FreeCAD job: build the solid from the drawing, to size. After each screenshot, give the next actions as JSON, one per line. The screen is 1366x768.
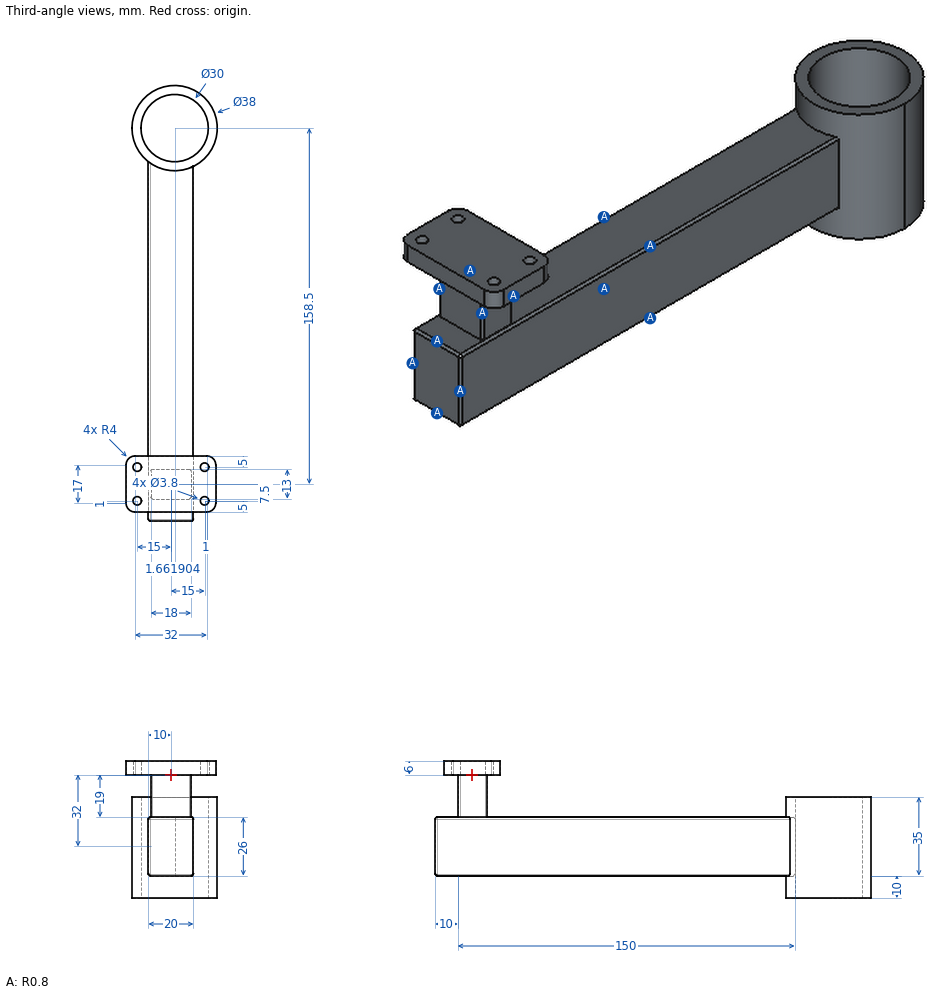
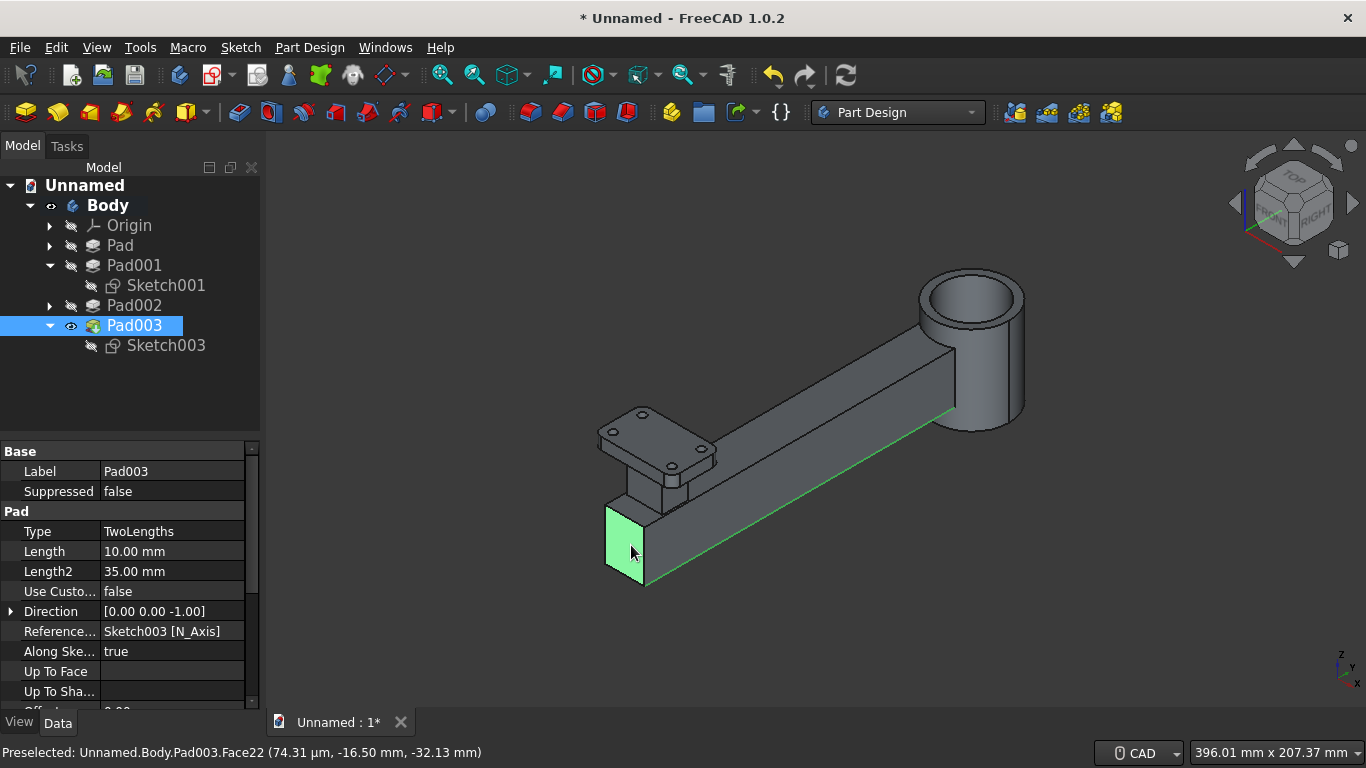
{"action": "left_click", "coordinate": [662, 492], "text": "ctrl"}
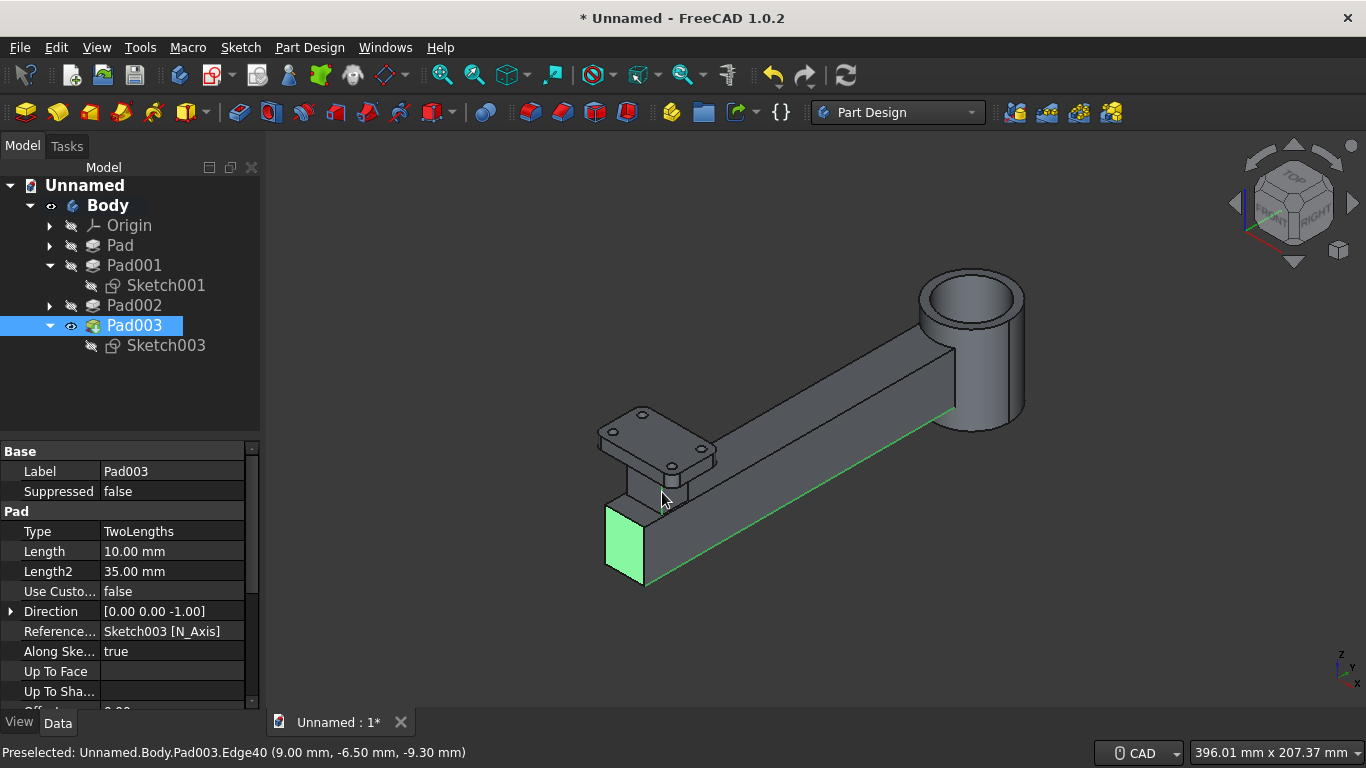
{"action": "left_click", "coordinate": [800, 437], "text": "ctrl"}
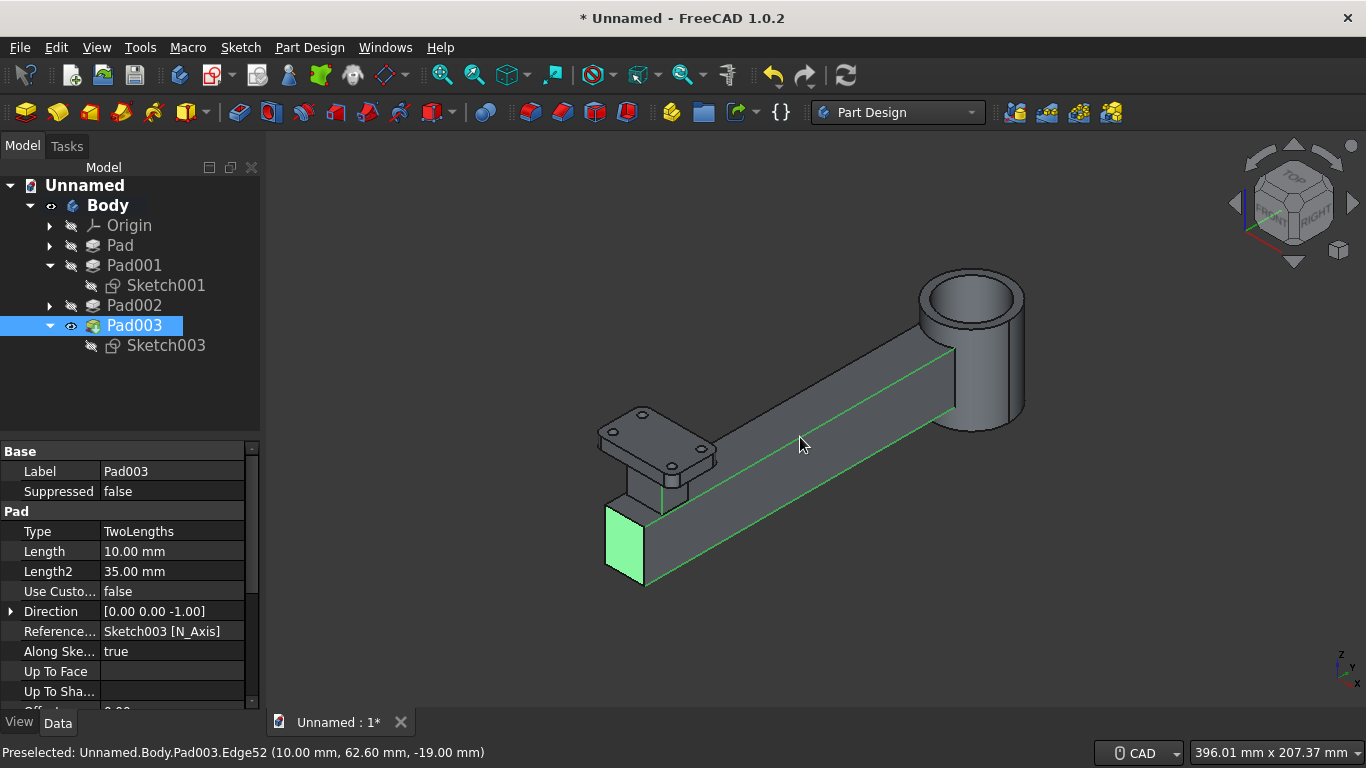
{"action": "key", "text": "2"}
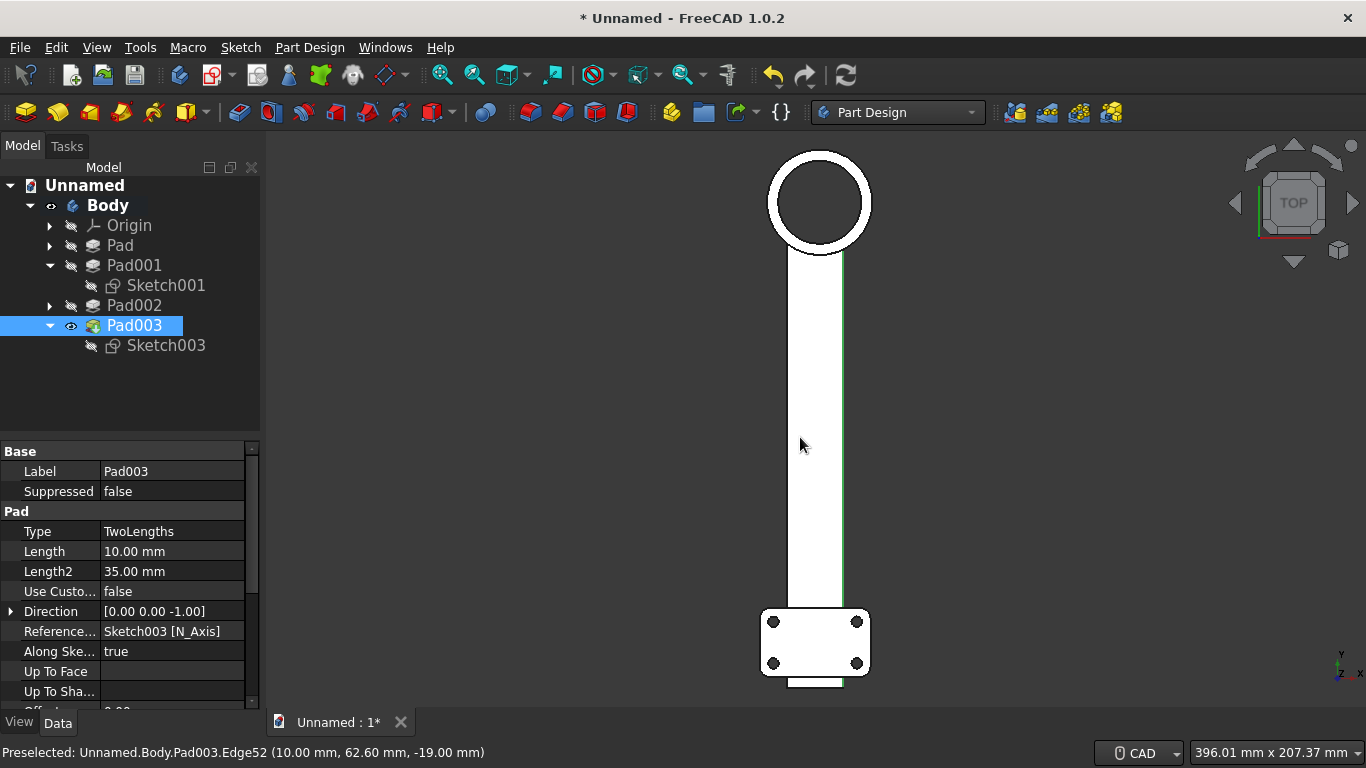
{"action": "left_click", "coordinate": [787, 465], "text": "ctrl"}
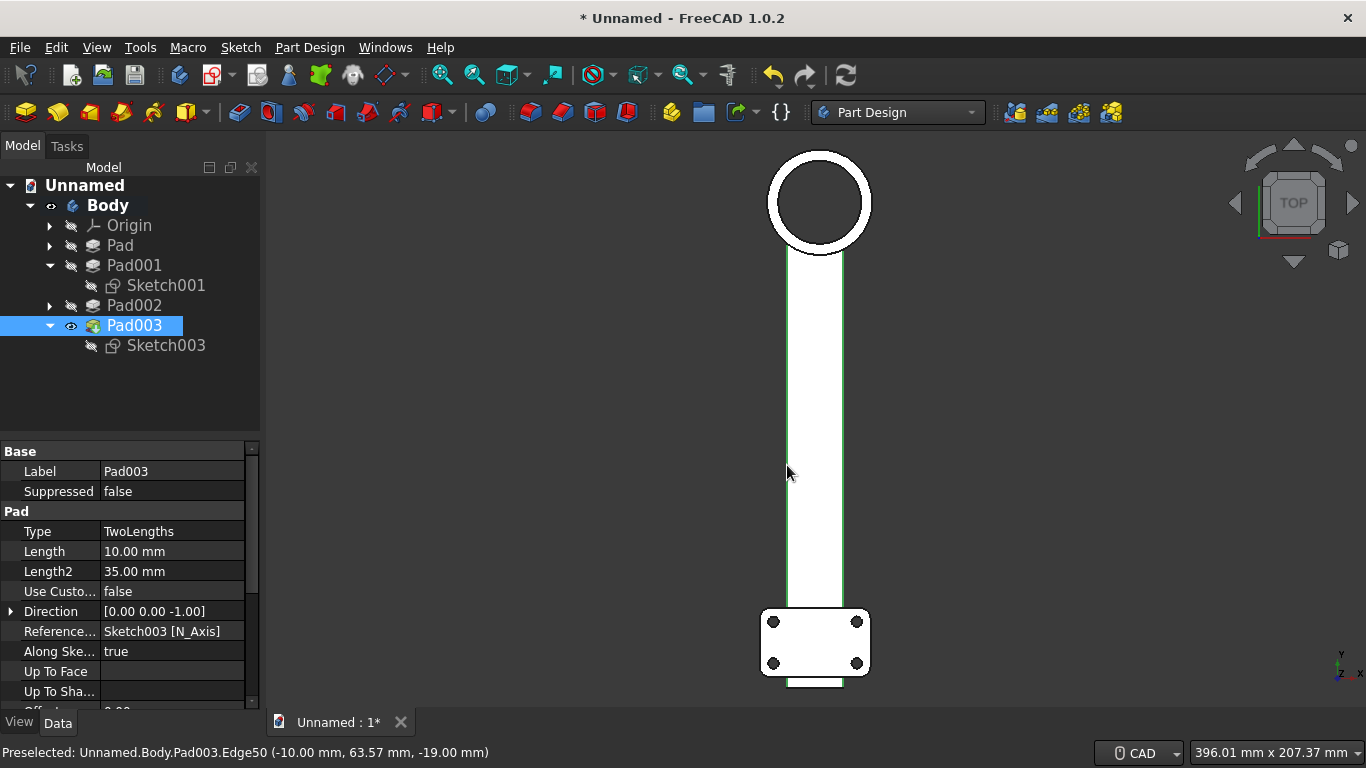
{"action": "key", "text": "1"}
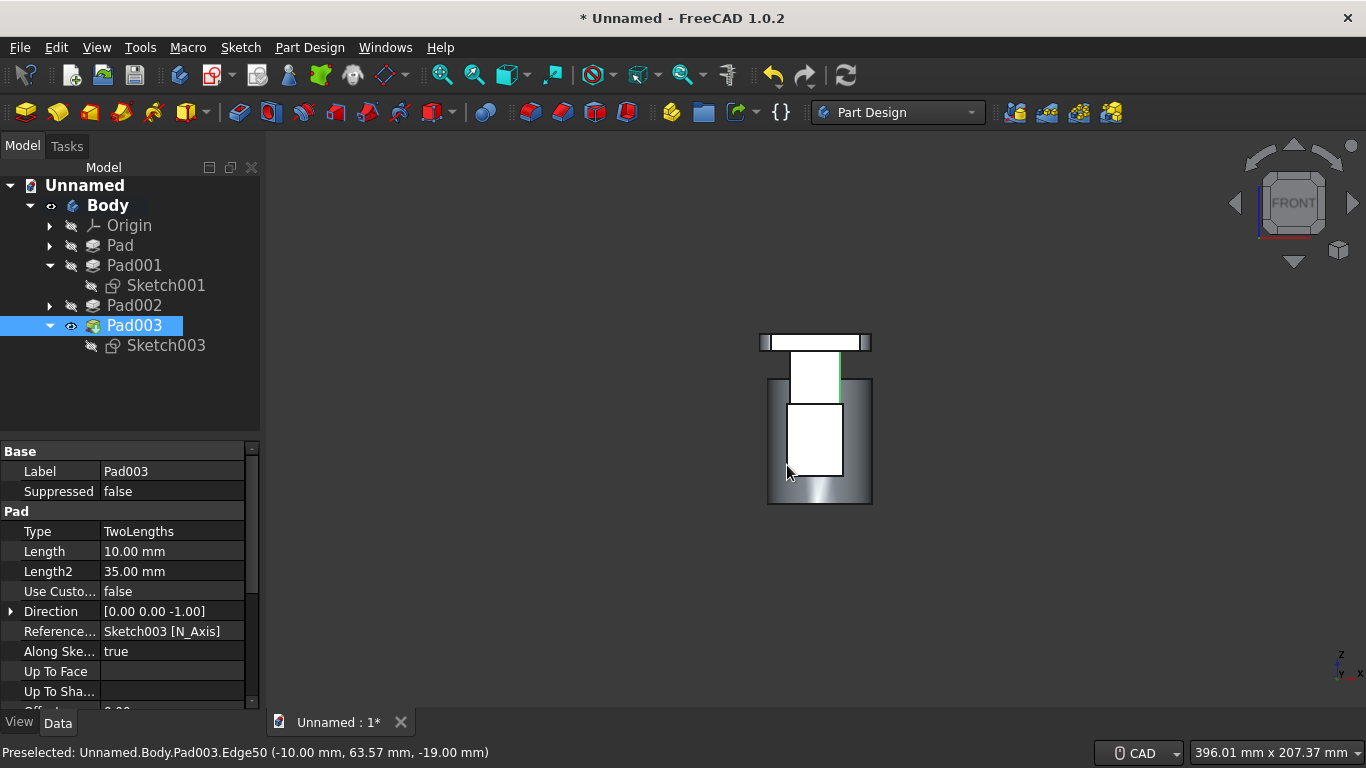
{"action": "left_click", "coordinate": [444, 76]}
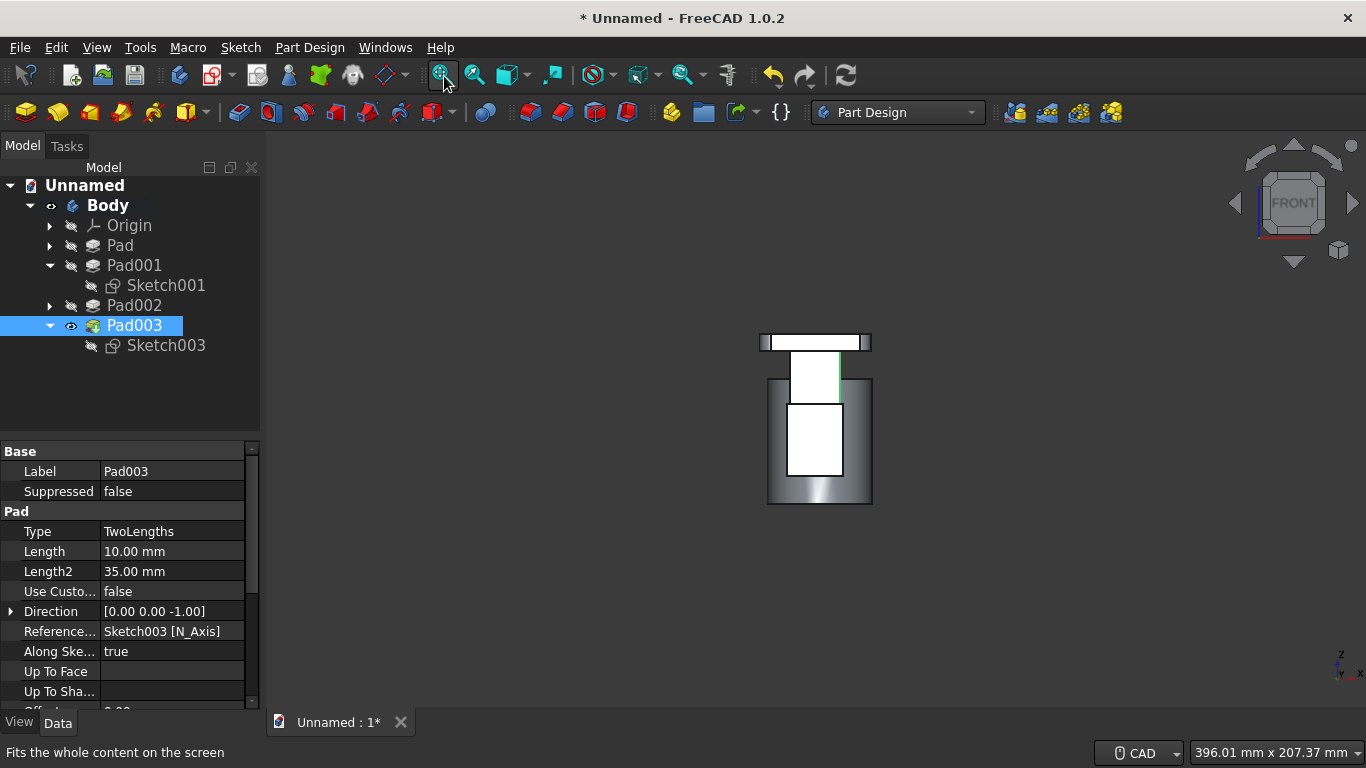
{"action": "left_click", "coordinate": [790, 376], "text": "ctrl"}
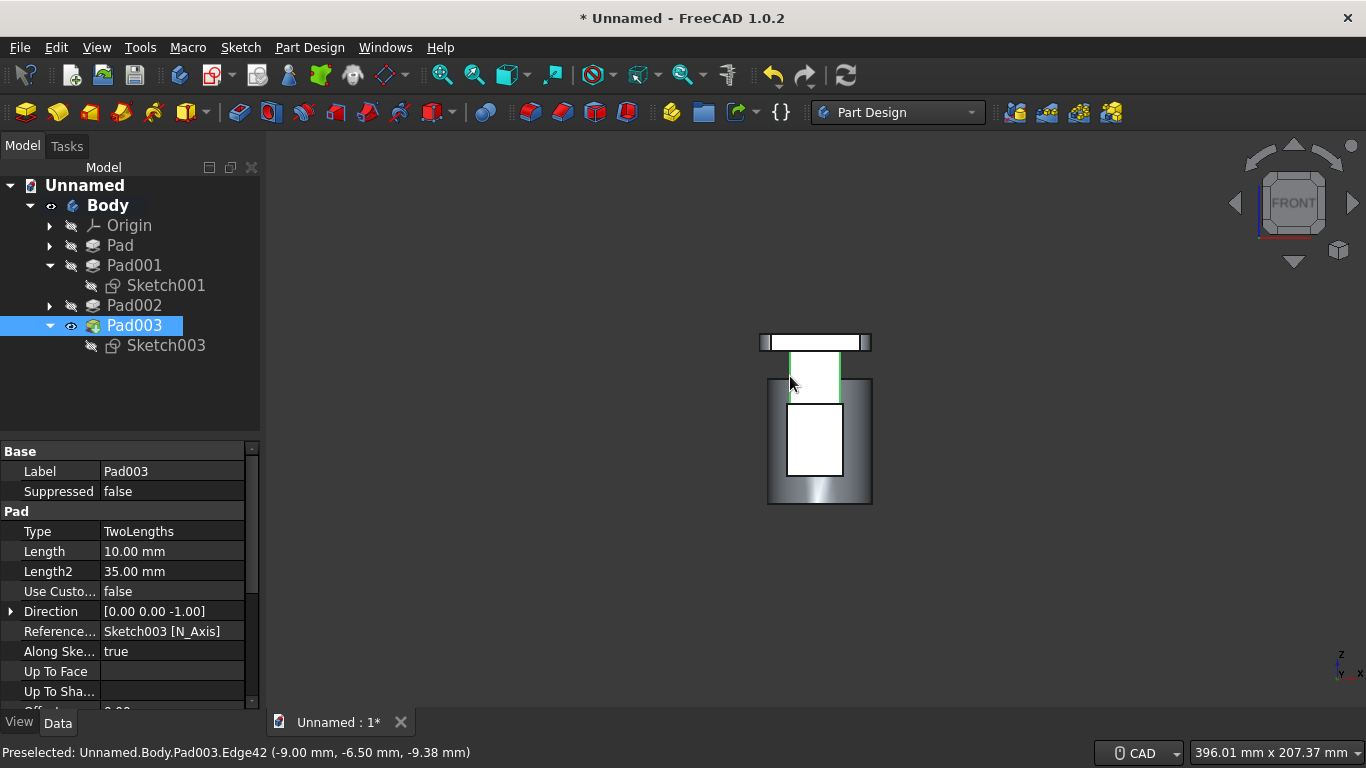
{"action": "key", "text": "3"}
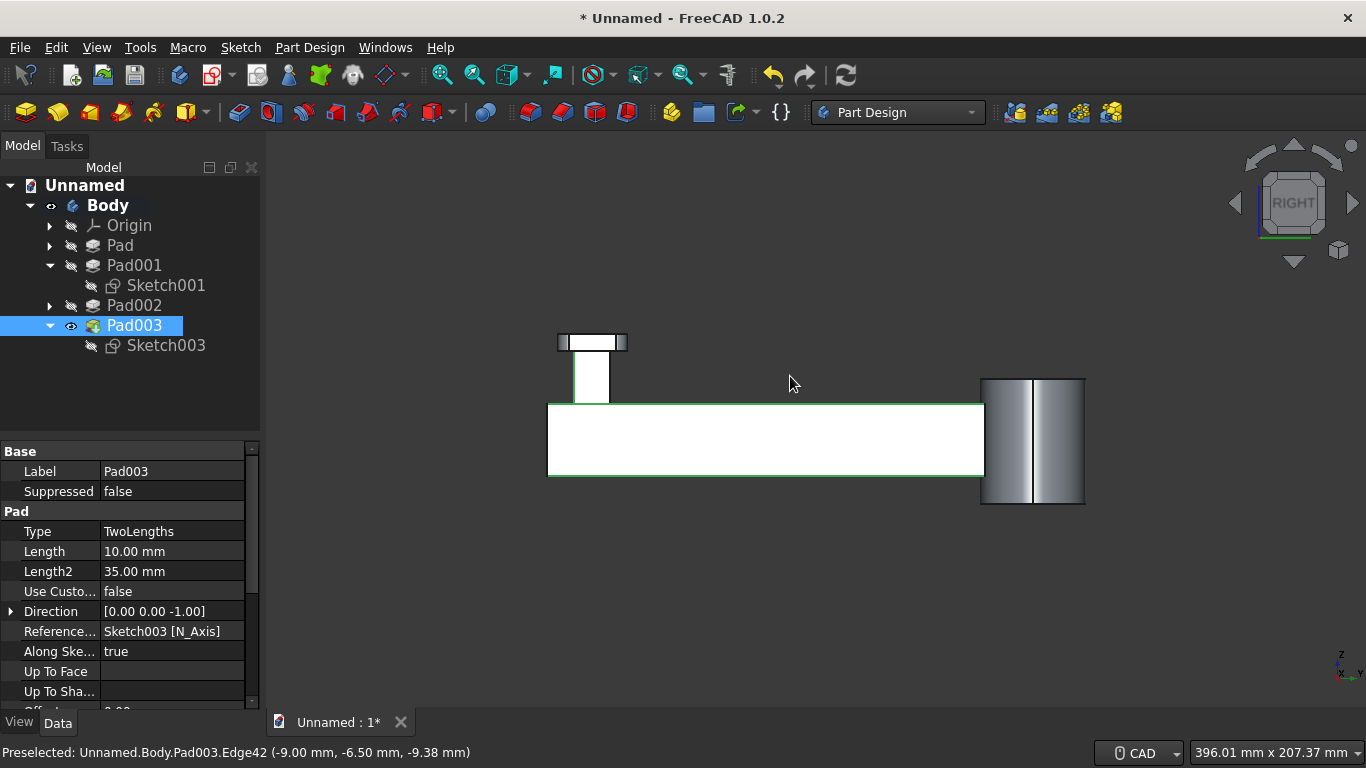
{"action": "left_click", "coordinate": [610, 376], "text": "ctrl"}